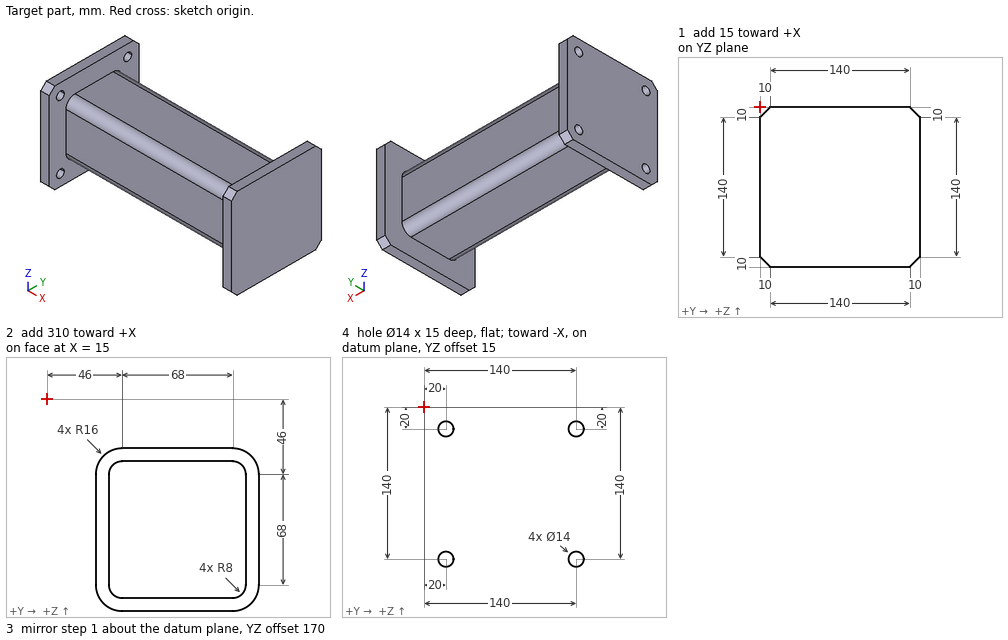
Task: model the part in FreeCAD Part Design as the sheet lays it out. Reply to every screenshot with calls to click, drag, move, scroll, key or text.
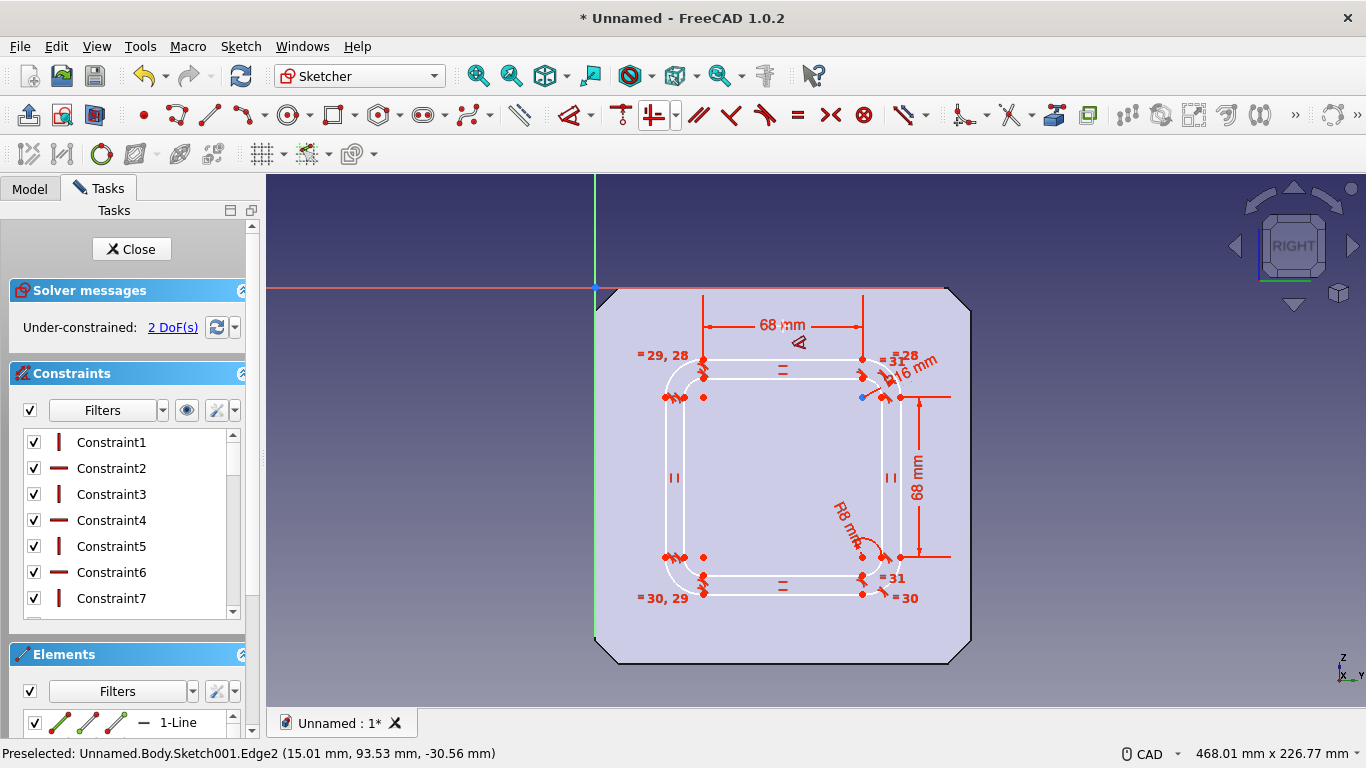
click(901, 397)
click(561, 343)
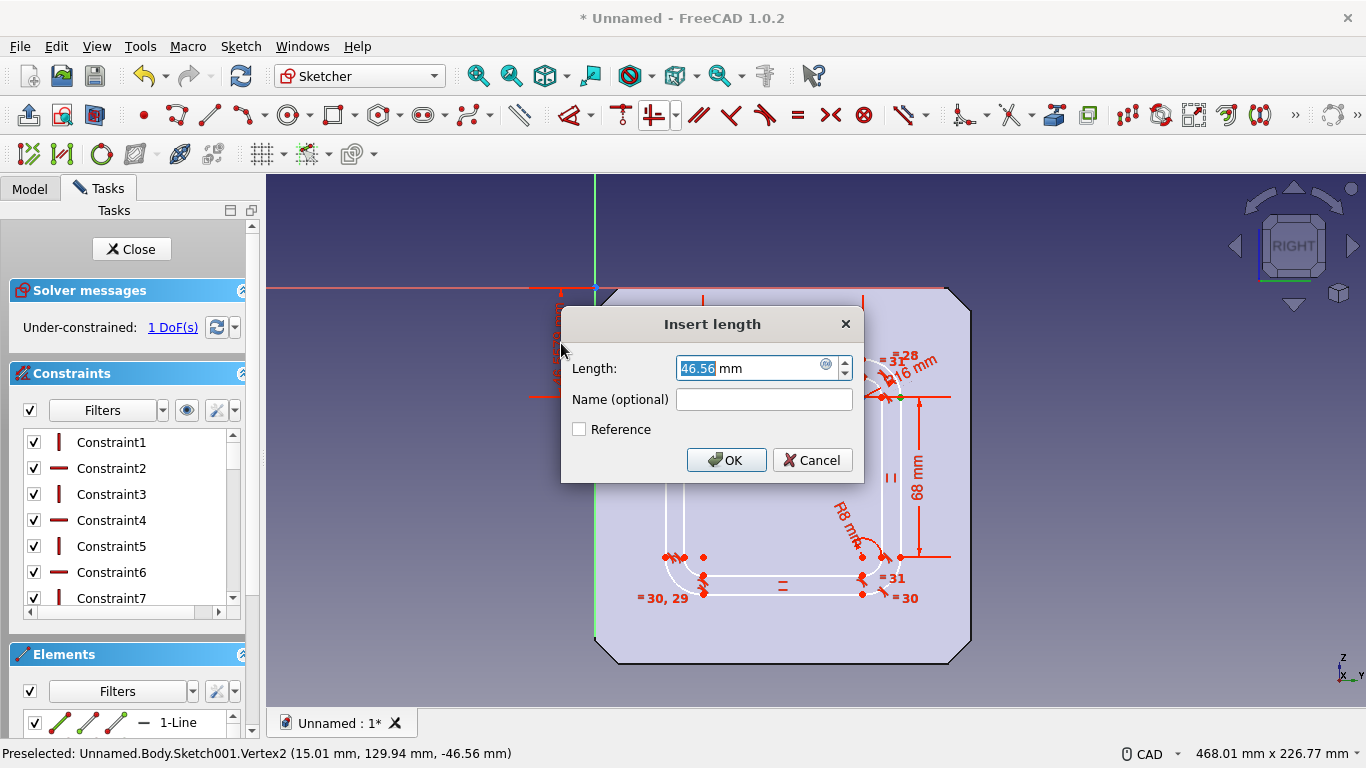
text(46)
key(Return)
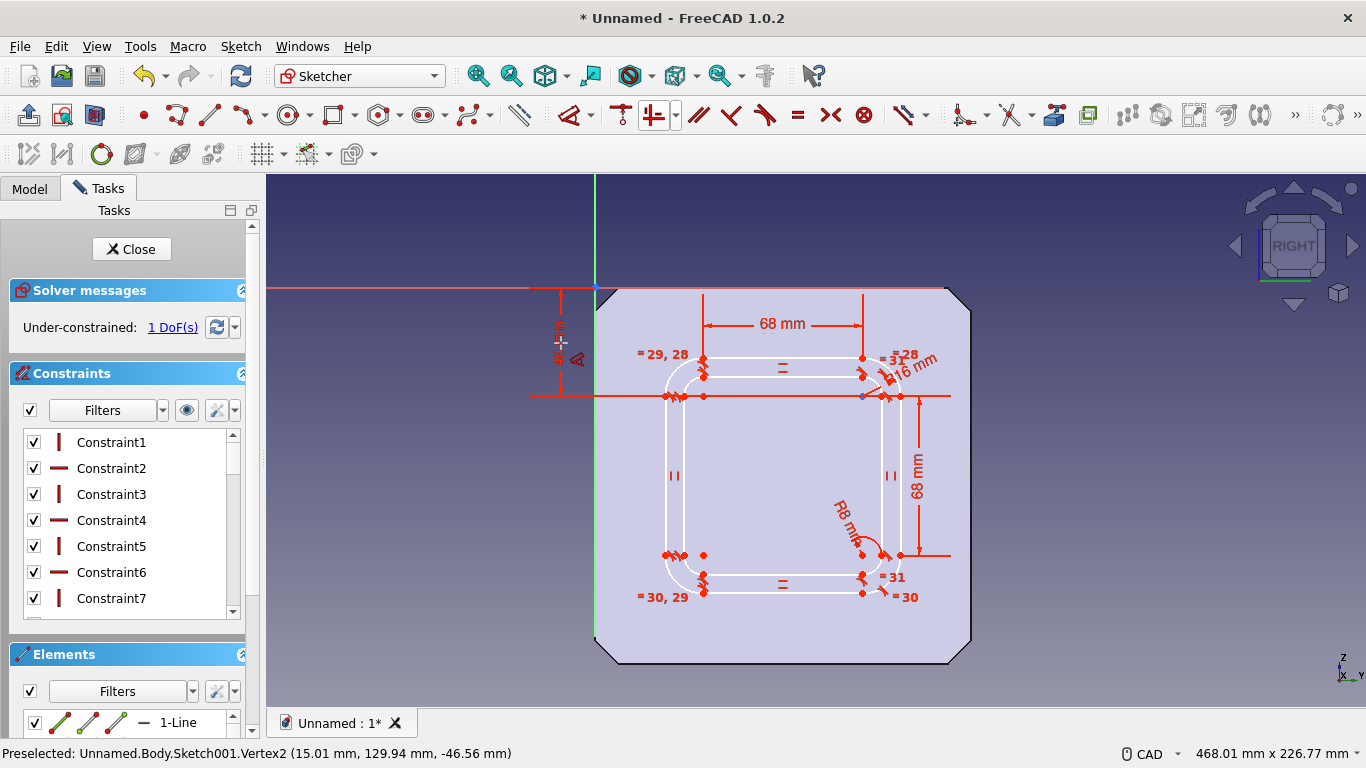
click(703, 358)
click(649, 254)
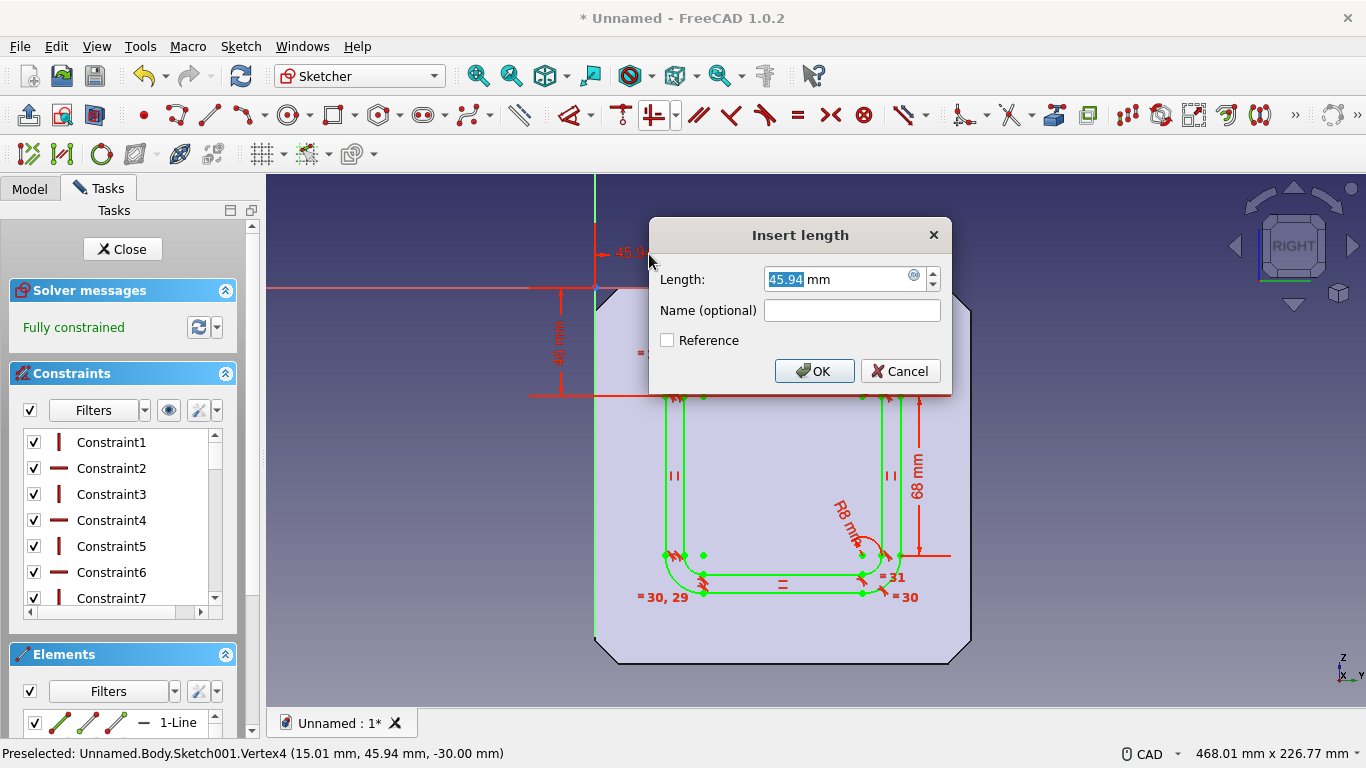
text(46)
key(Return)
key(Escape)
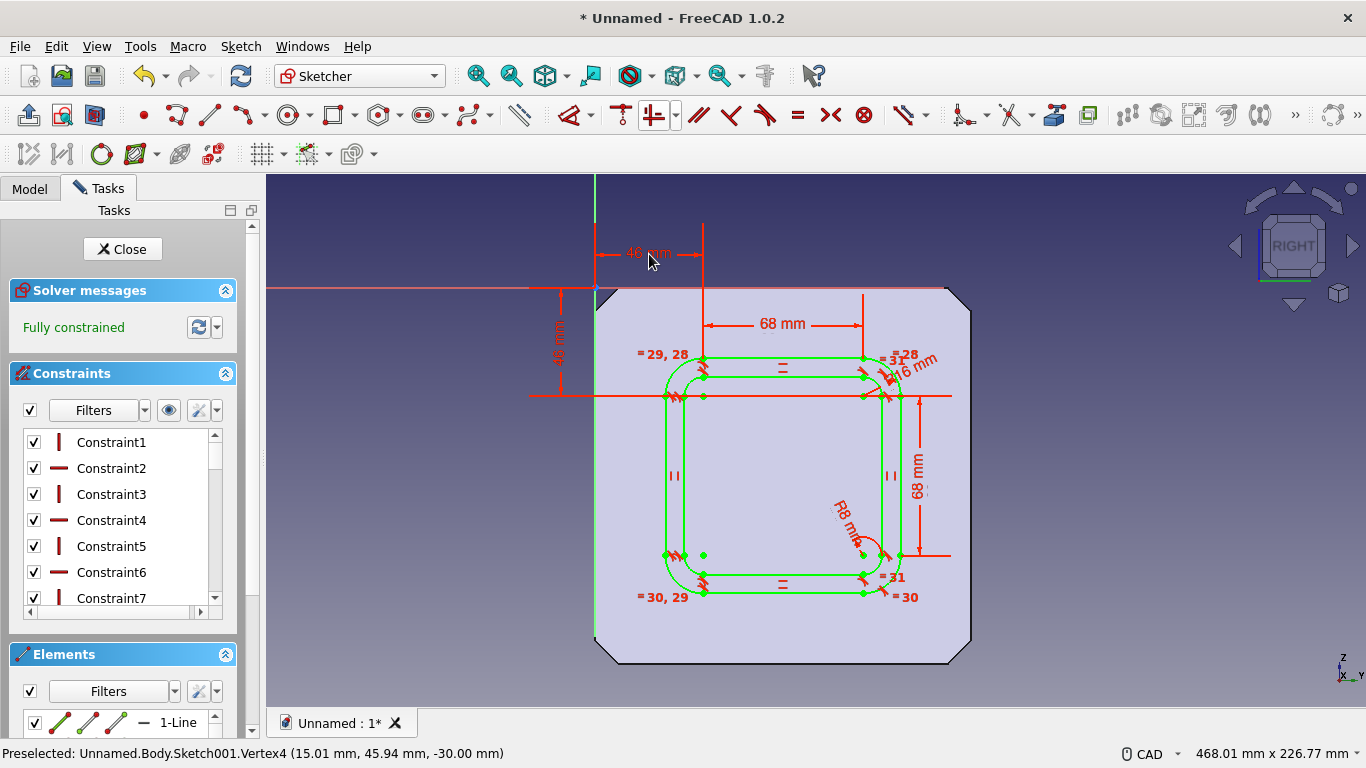
click(123, 249)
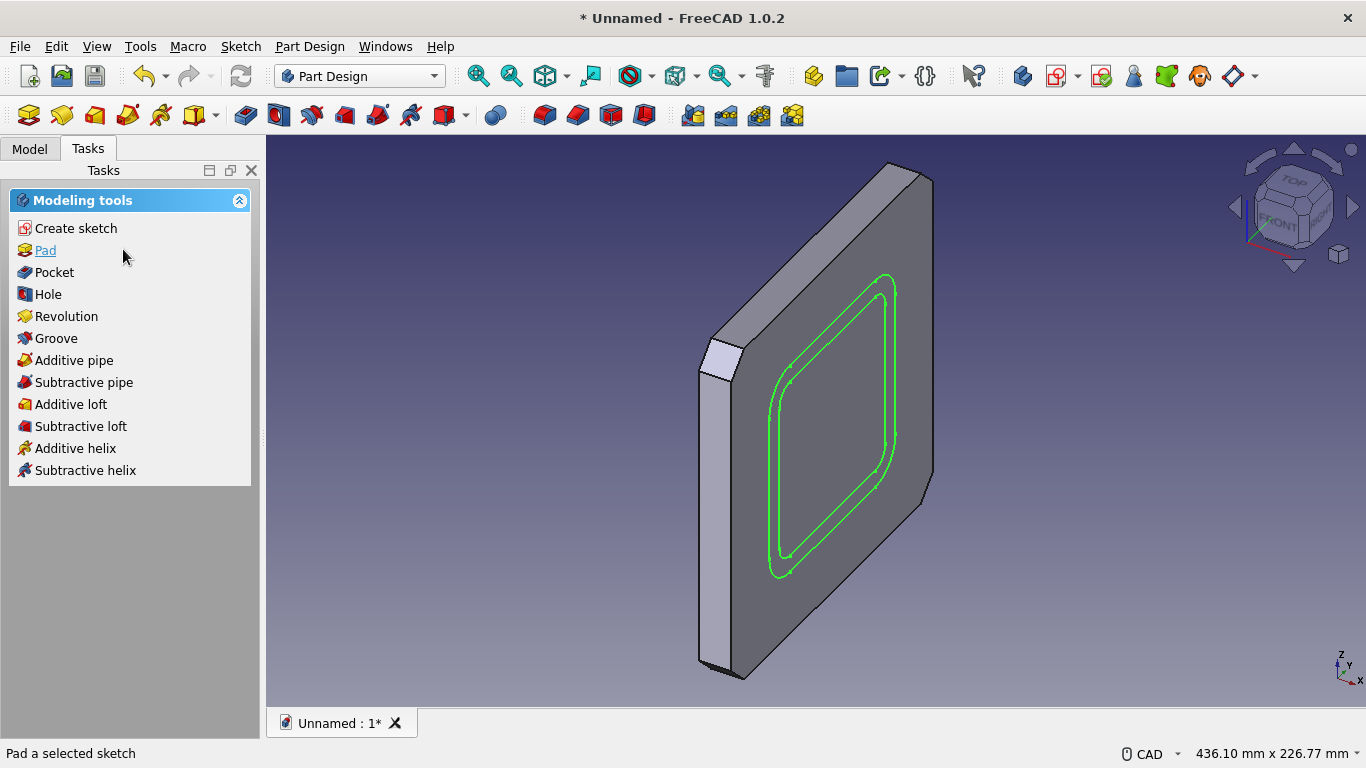
click(29, 116)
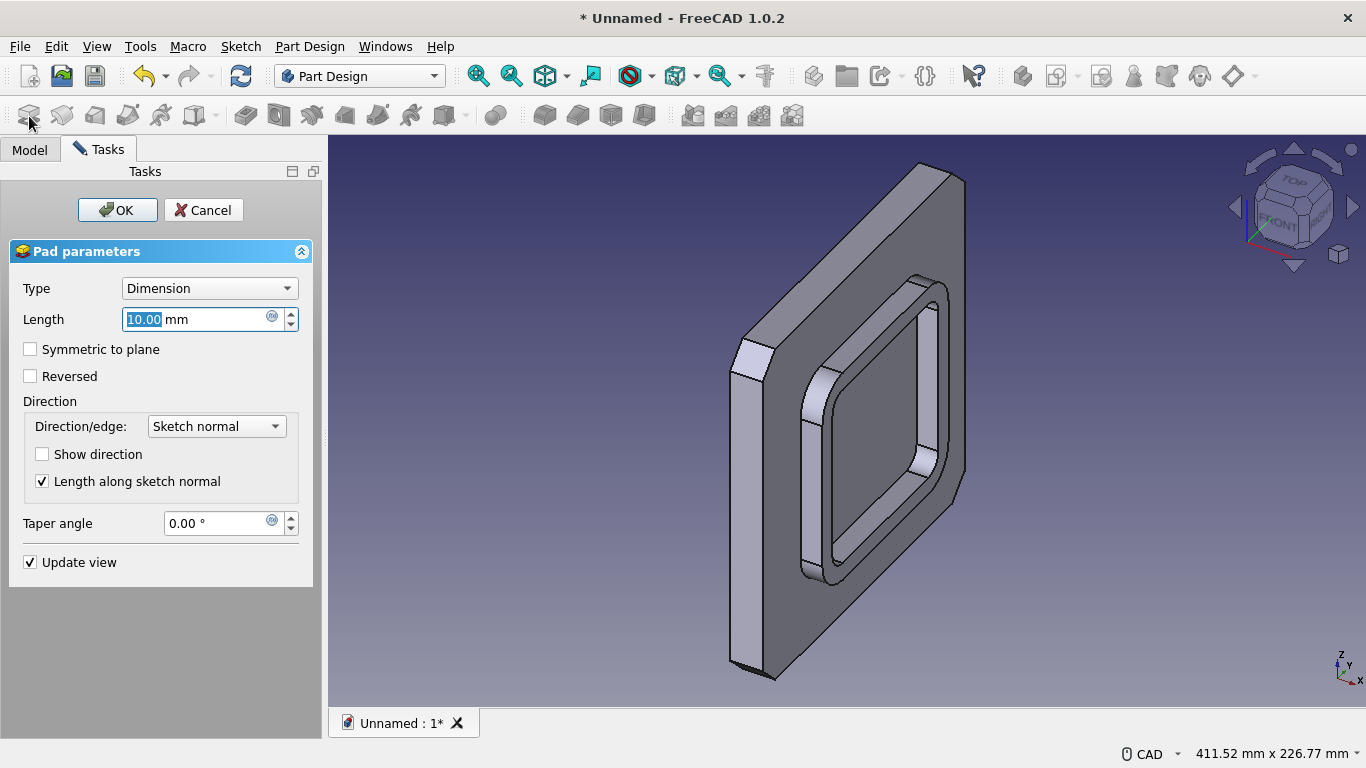
text(310)
key(Tab)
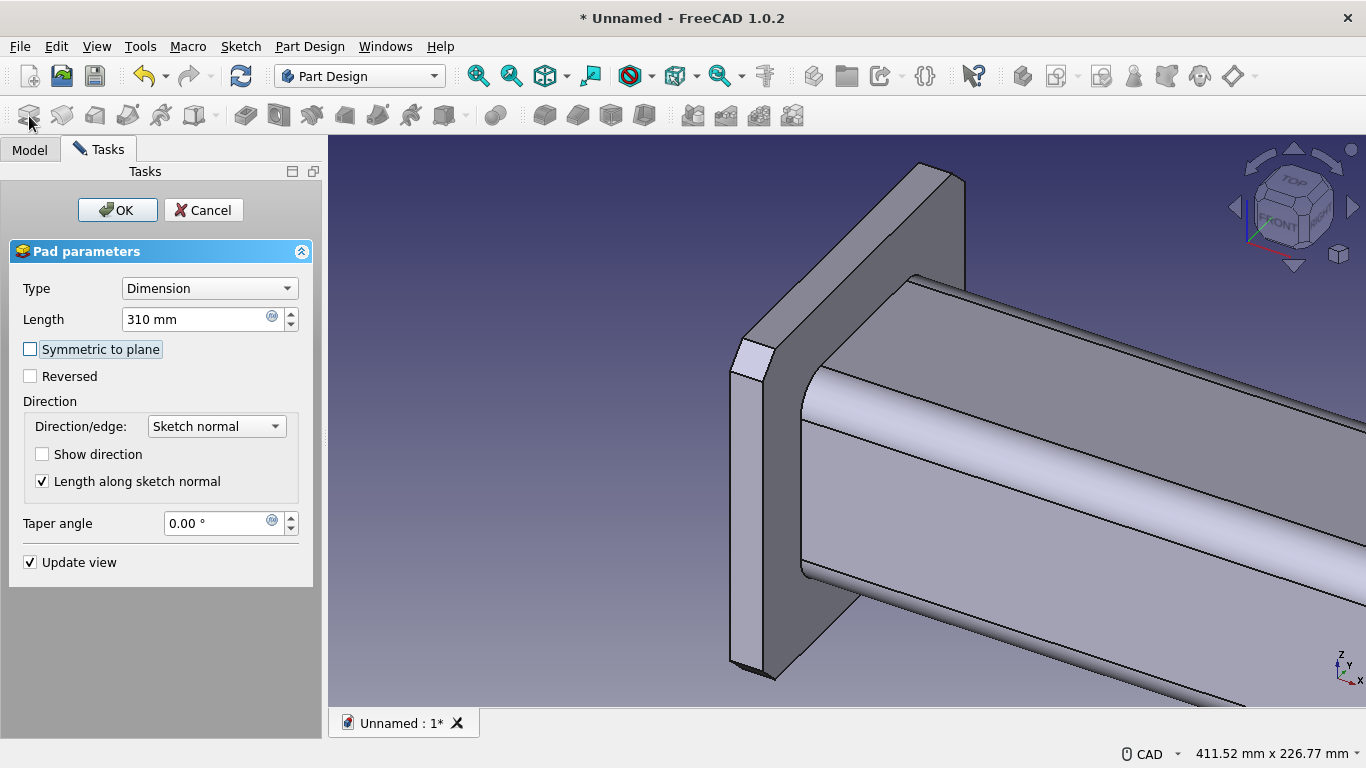
click(118, 210)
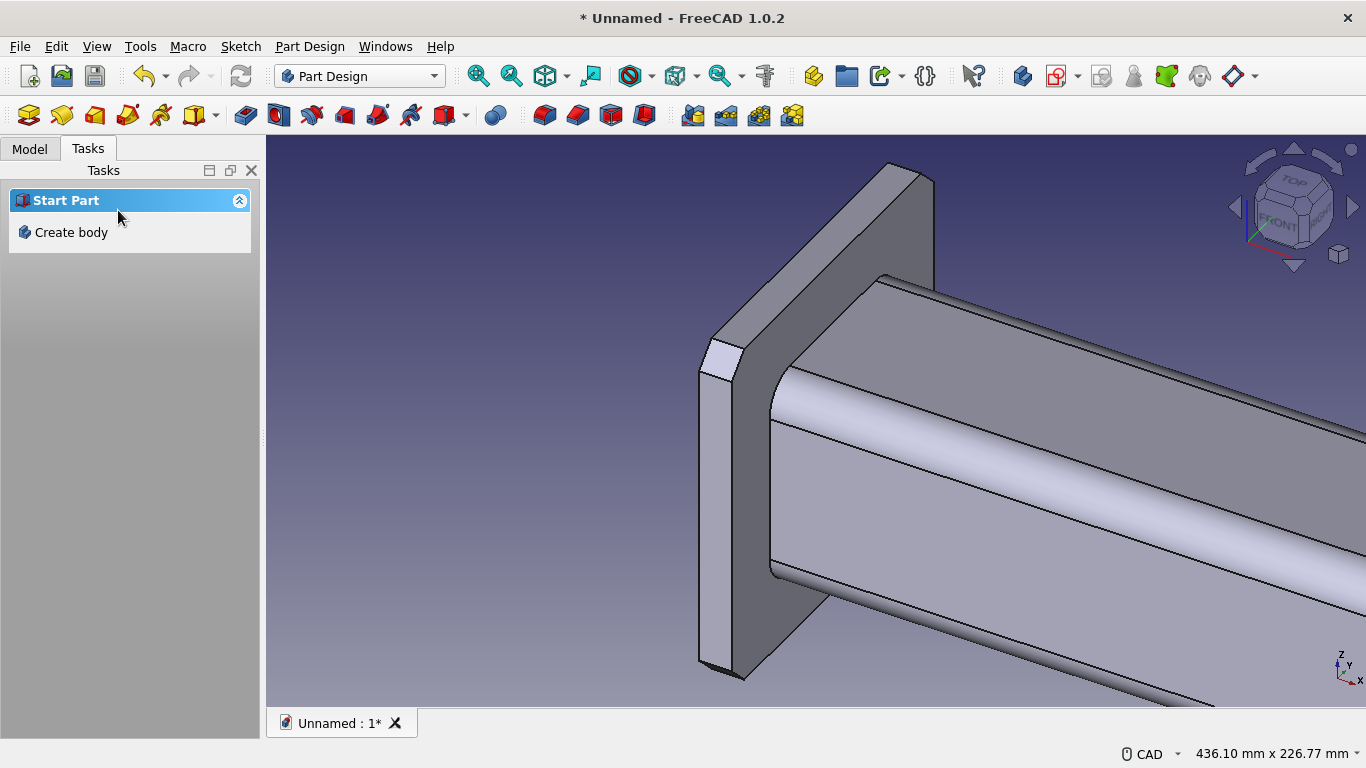
click(479, 76)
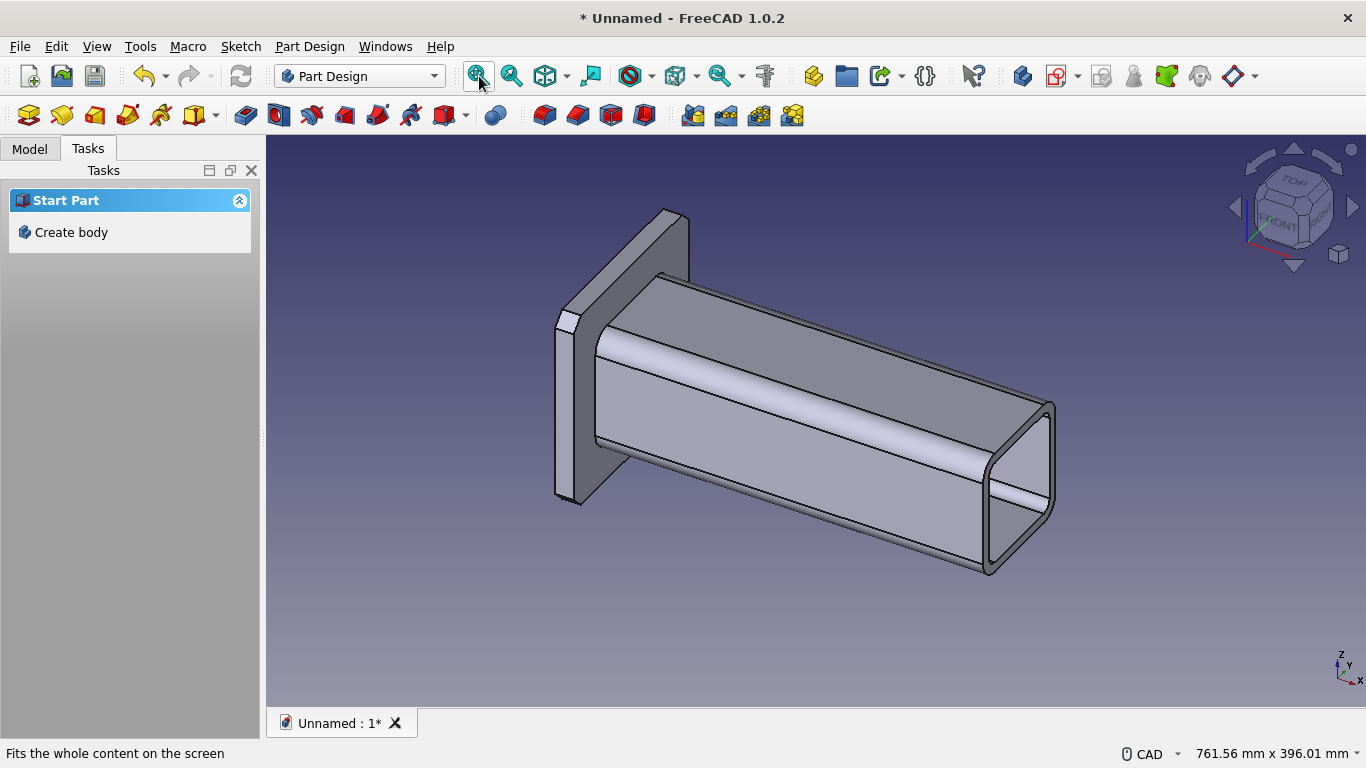
click(30, 148)